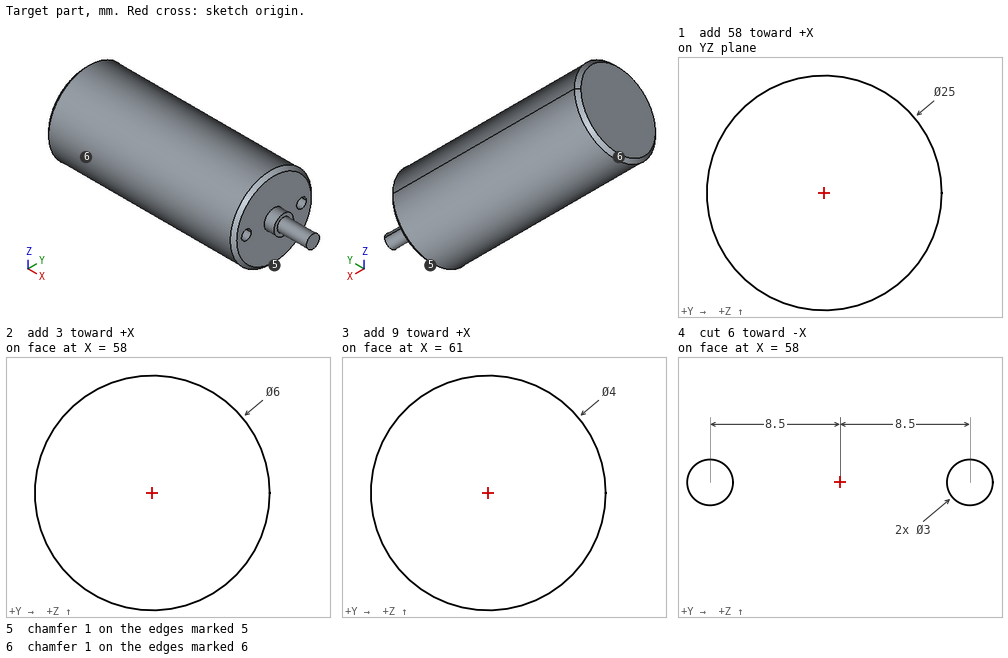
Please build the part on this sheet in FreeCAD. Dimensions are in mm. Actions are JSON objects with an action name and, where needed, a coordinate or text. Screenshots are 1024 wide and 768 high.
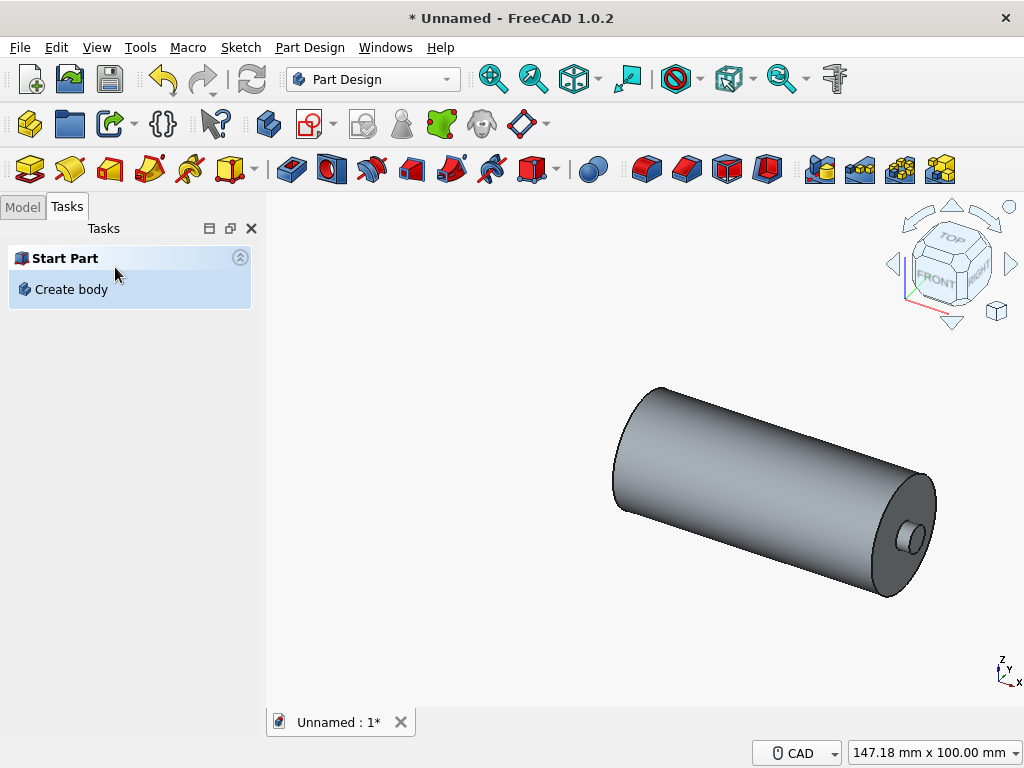
{"action": "key", "text": "0"}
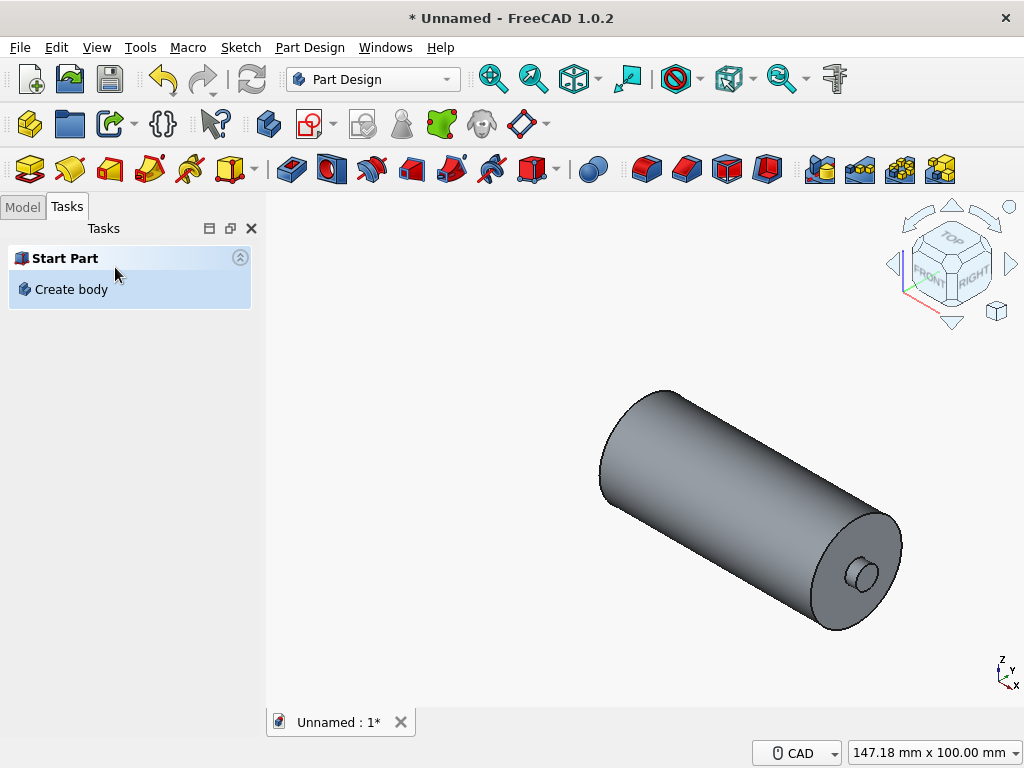
{"action": "left_click", "coordinate": [870, 575]}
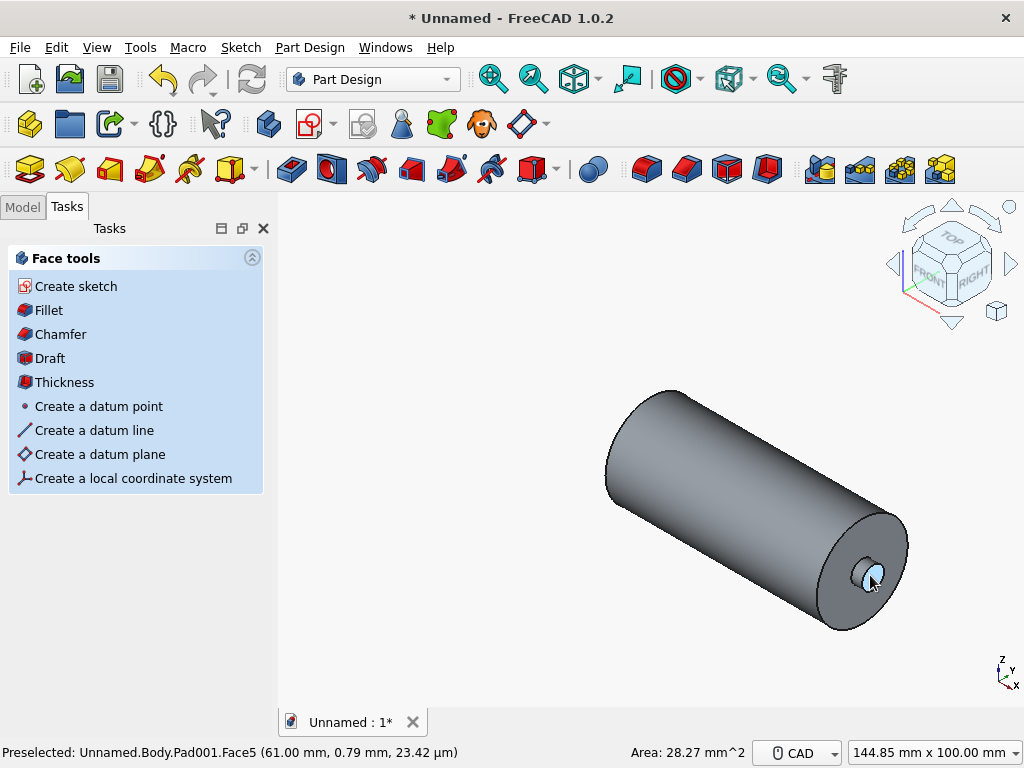
{"action": "left_click", "coordinate": [310, 124]}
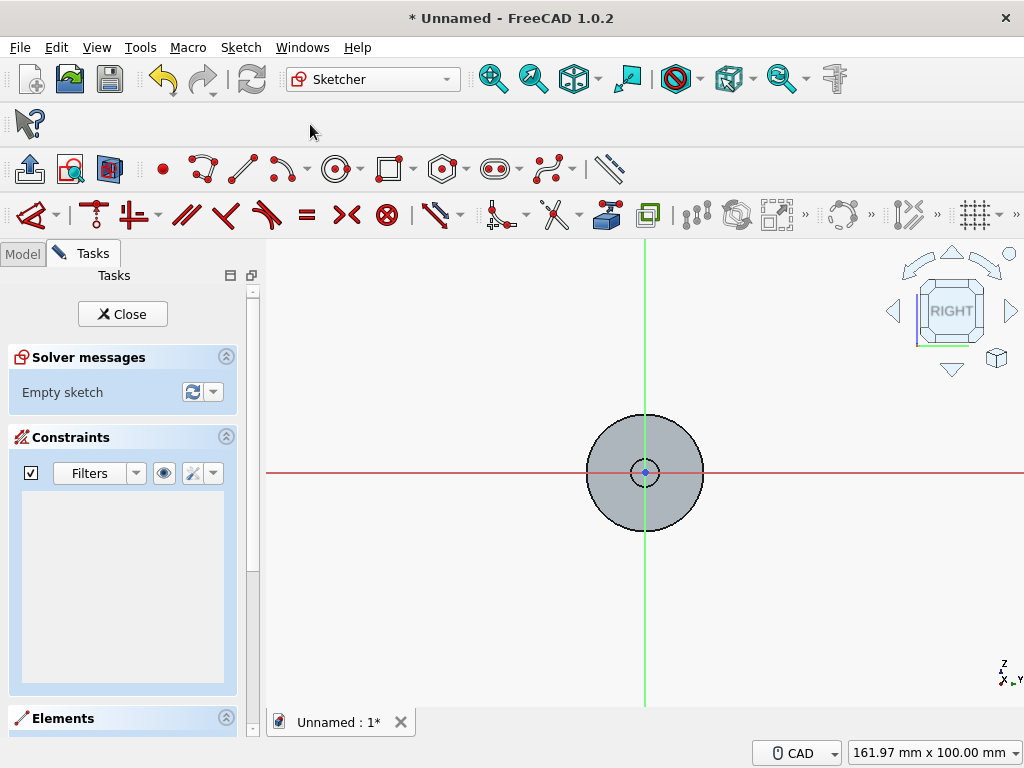
{"action": "scroll", "coordinate": [649, 473], "scroll_direction": "up", "scroll_amount": 14}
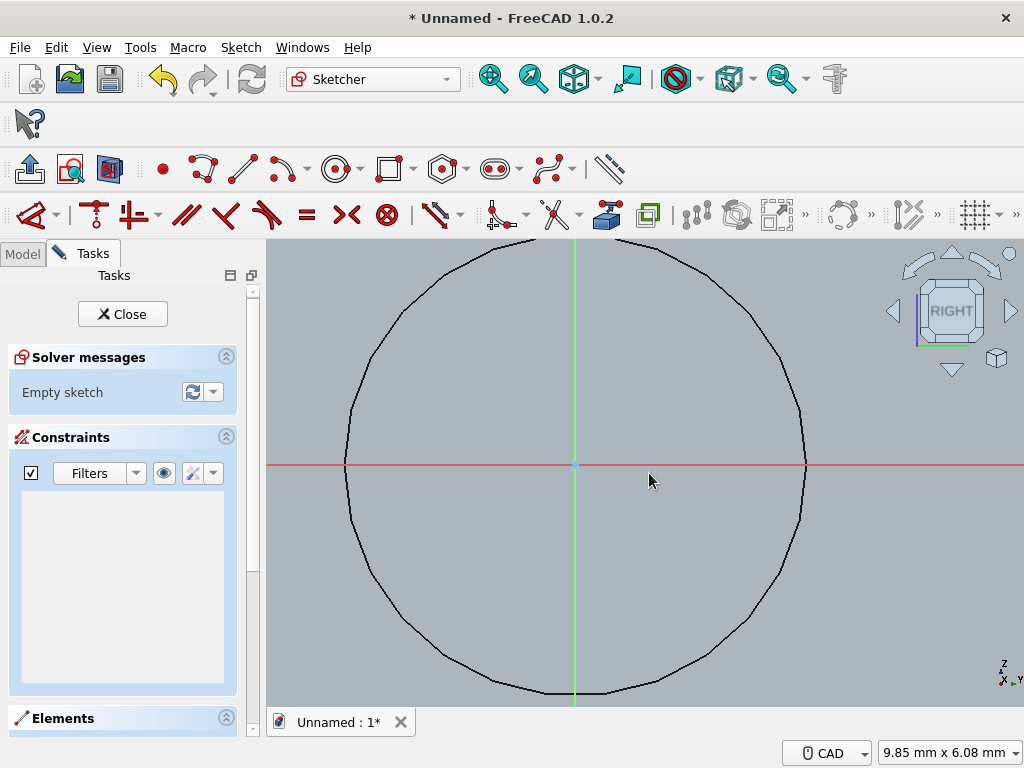
{"action": "key", "text": "g c"}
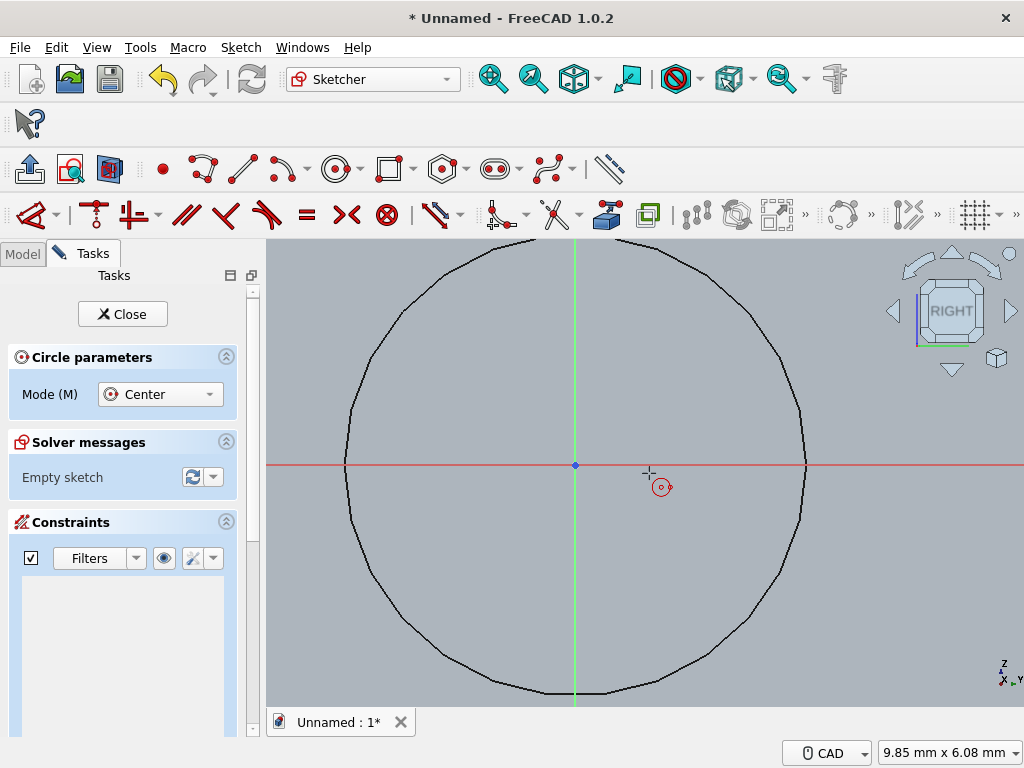
{"action": "left_click", "coordinate": [575, 465]}
{"action": "left_click", "coordinate": [684, 356]}
{"action": "key", "text": "Escape"}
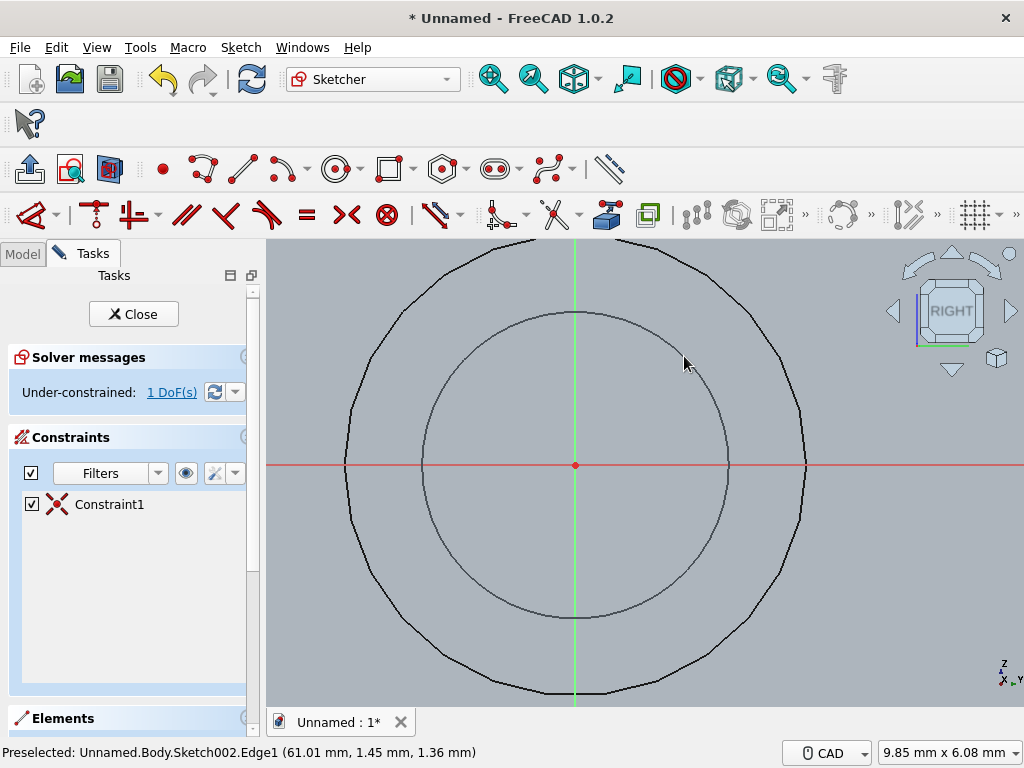
{"action": "left_click", "coordinate": [32, 216]}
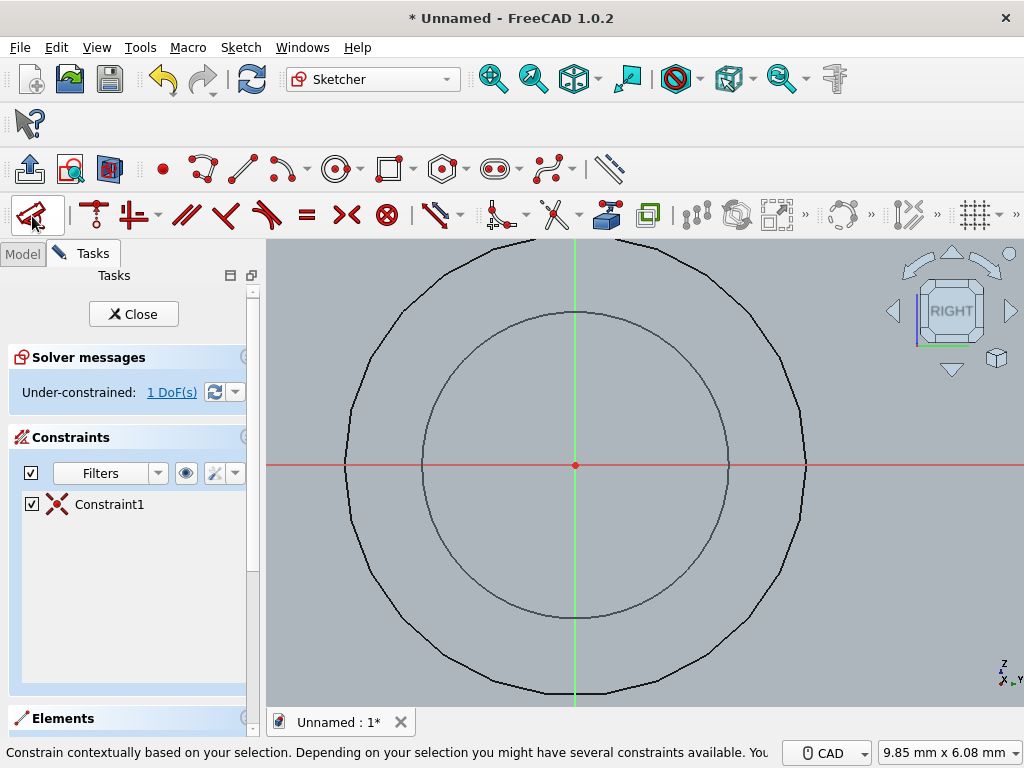
{"action": "left_click", "coordinate": [683, 356]}
{"action": "left_click", "coordinate": [705, 333]}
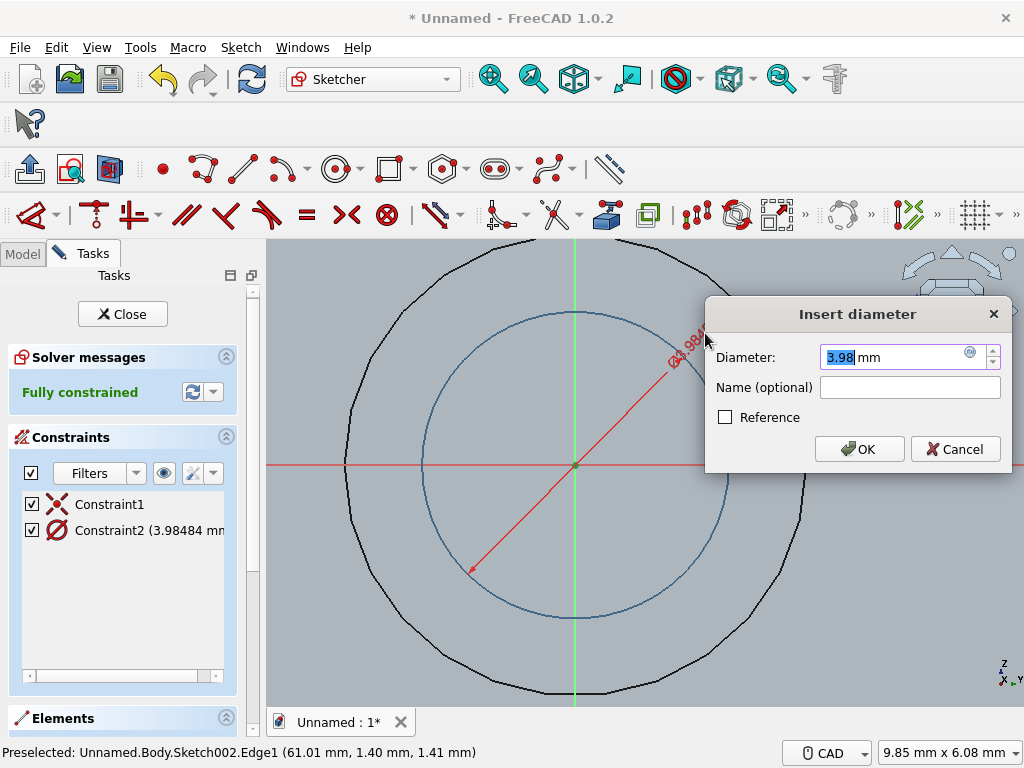
{"action": "type", "text": "4"}
{"action": "key", "text": "Return"}
{"action": "key", "text": "Escape"}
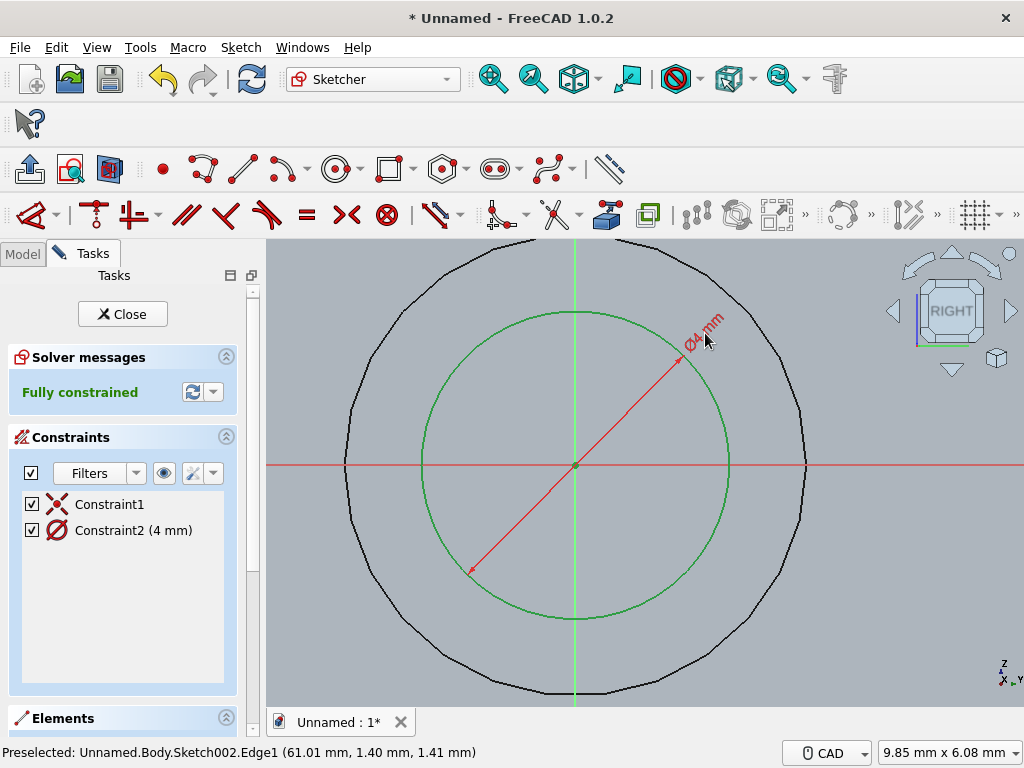
{"action": "left_click", "coordinate": [123, 314]}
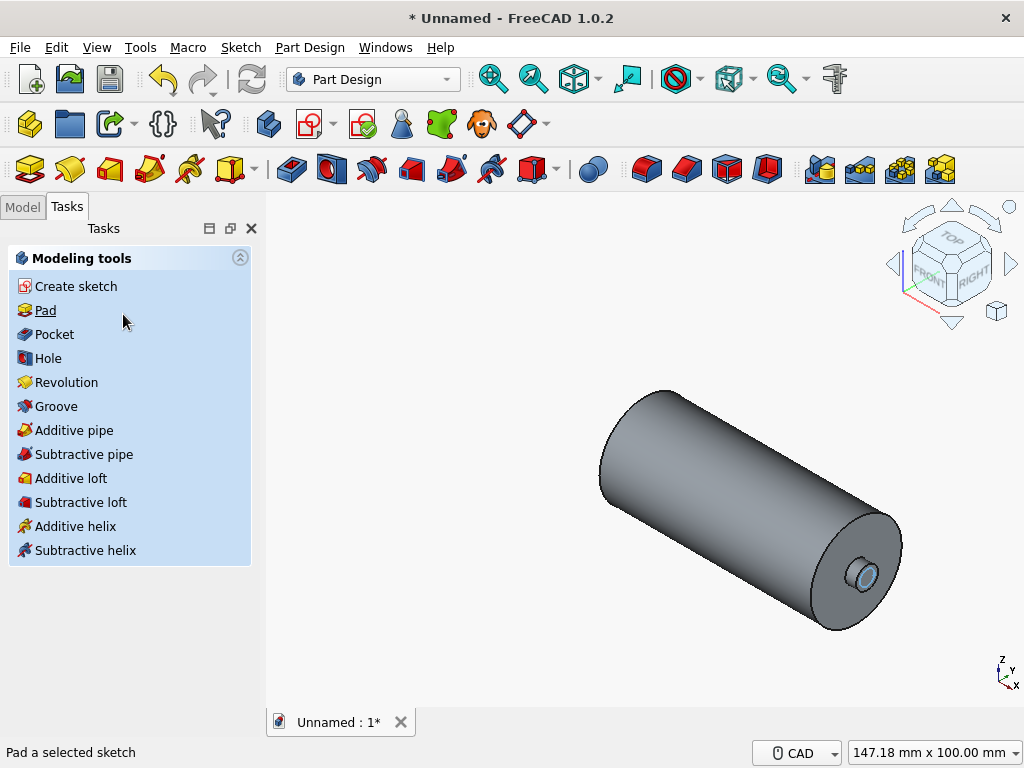
{"action": "left_click", "coordinate": [30, 170]}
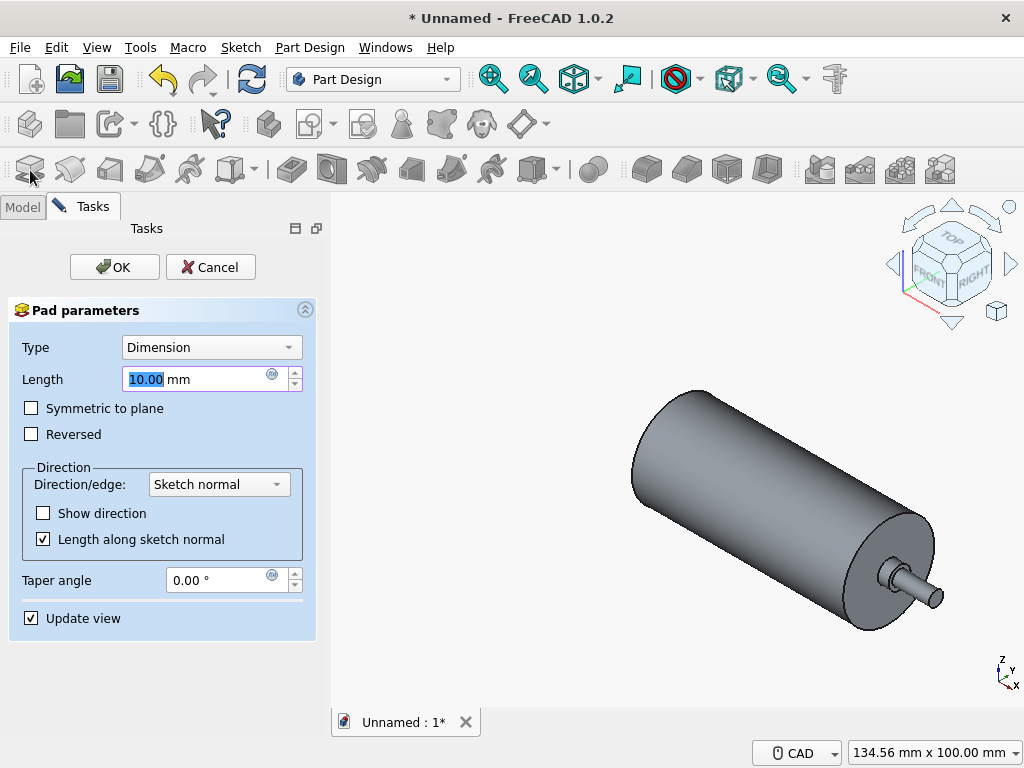
{"action": "type", "text": "9"}
{"action": "key", "text": "Tab"}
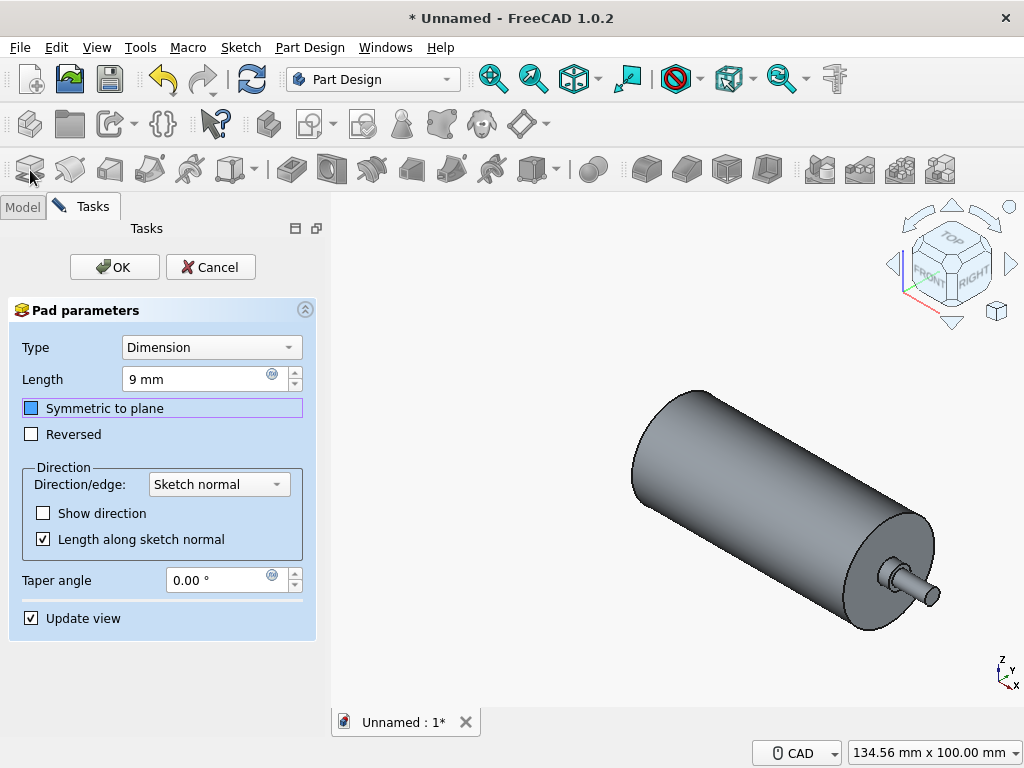
{"action": "left_click", "coordinate": [115, 267]}